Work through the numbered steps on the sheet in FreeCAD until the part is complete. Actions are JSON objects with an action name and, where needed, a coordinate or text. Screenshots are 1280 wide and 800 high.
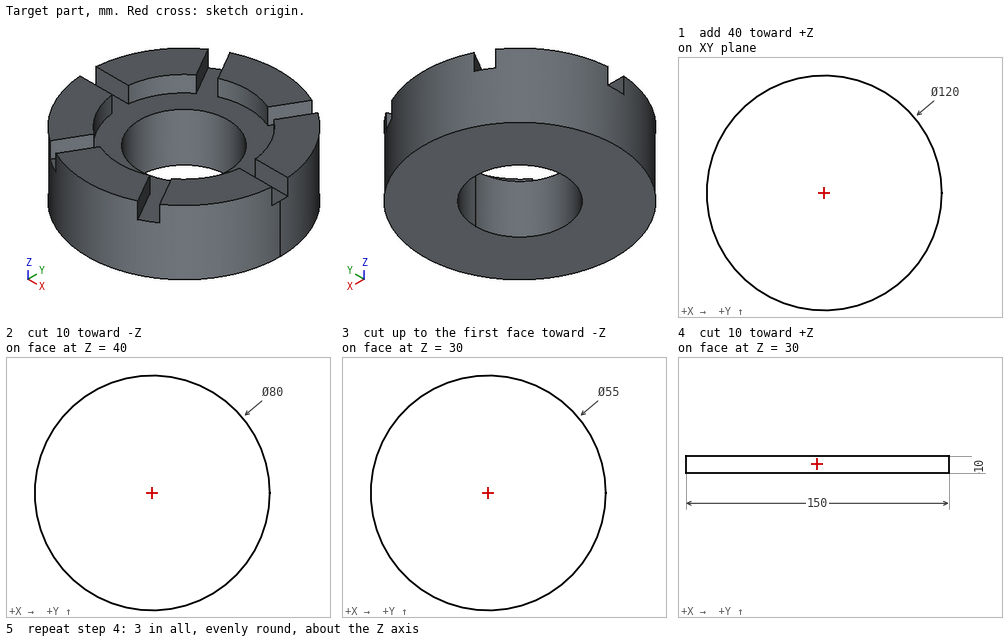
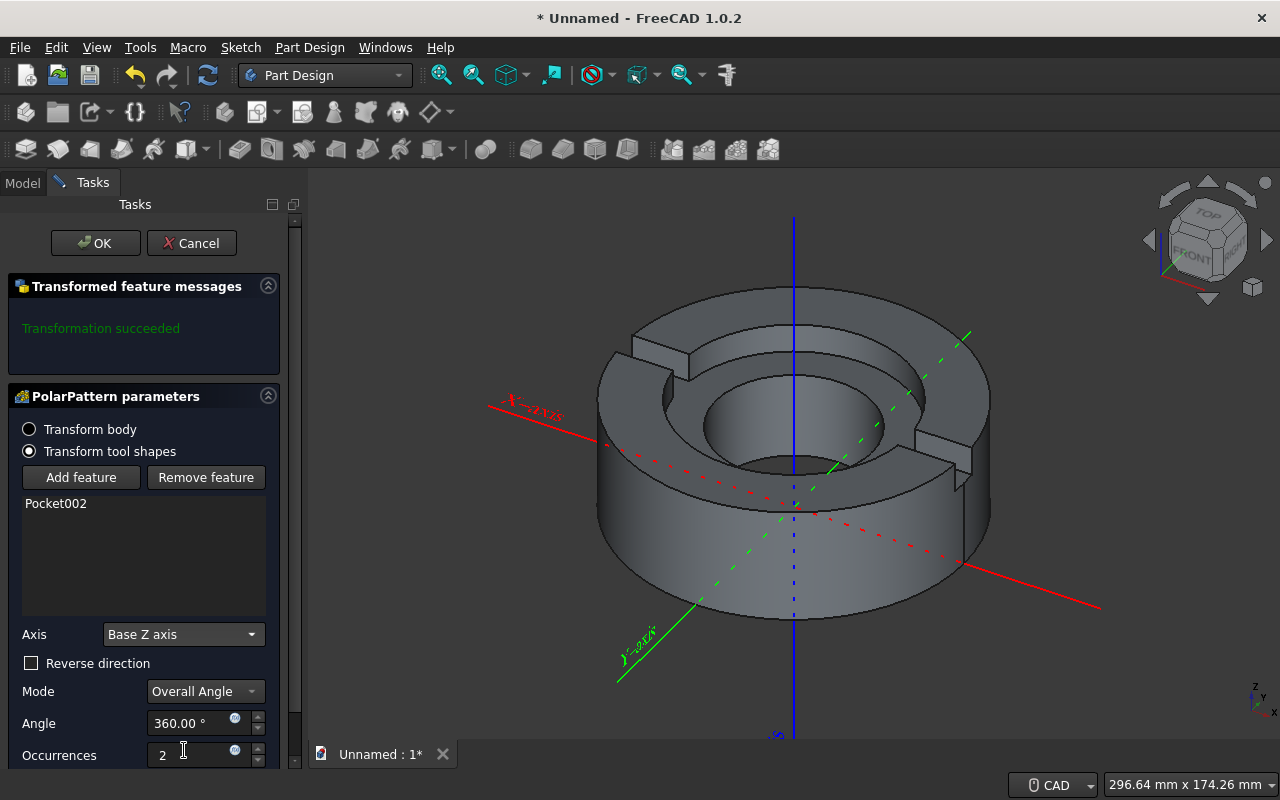
{"action": "triple_click", "coordinate": [198, 755]}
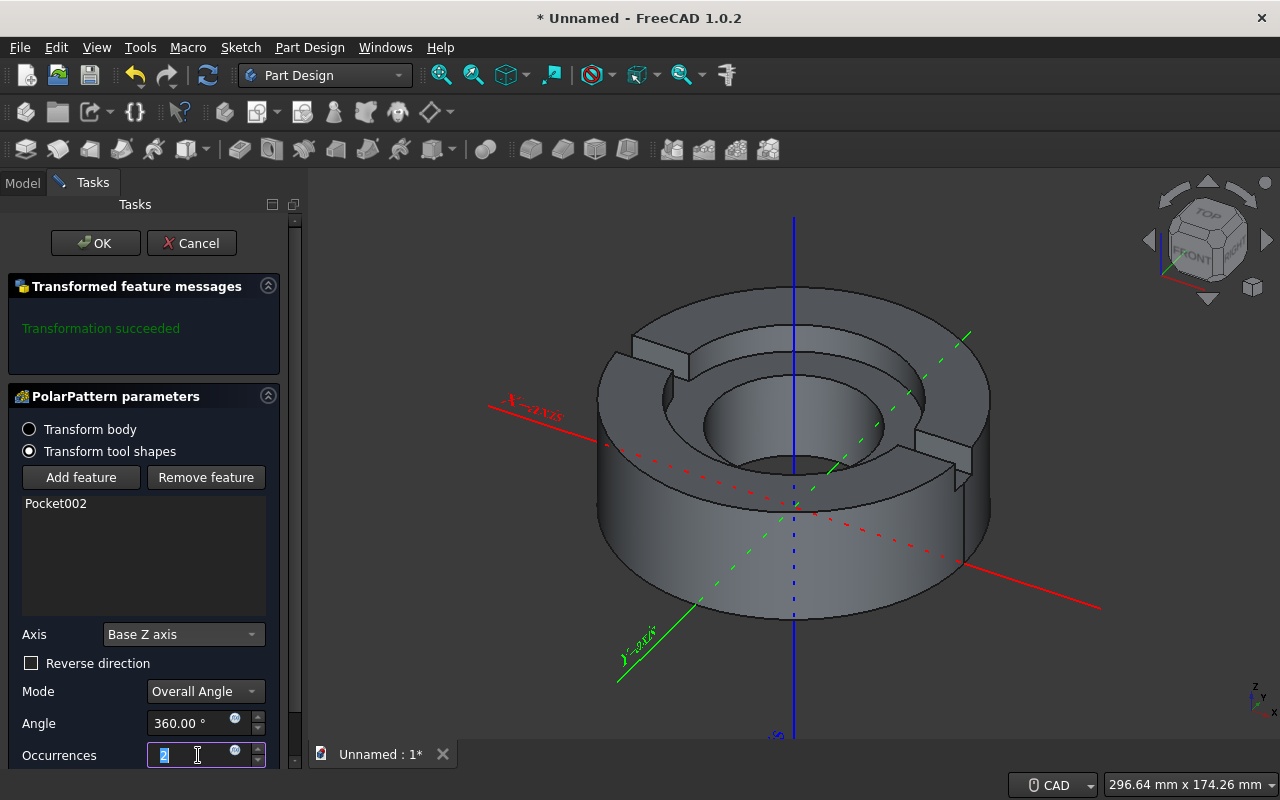
{"action": "type", "text": "3"}
{"action": "key", "text": "Tab"}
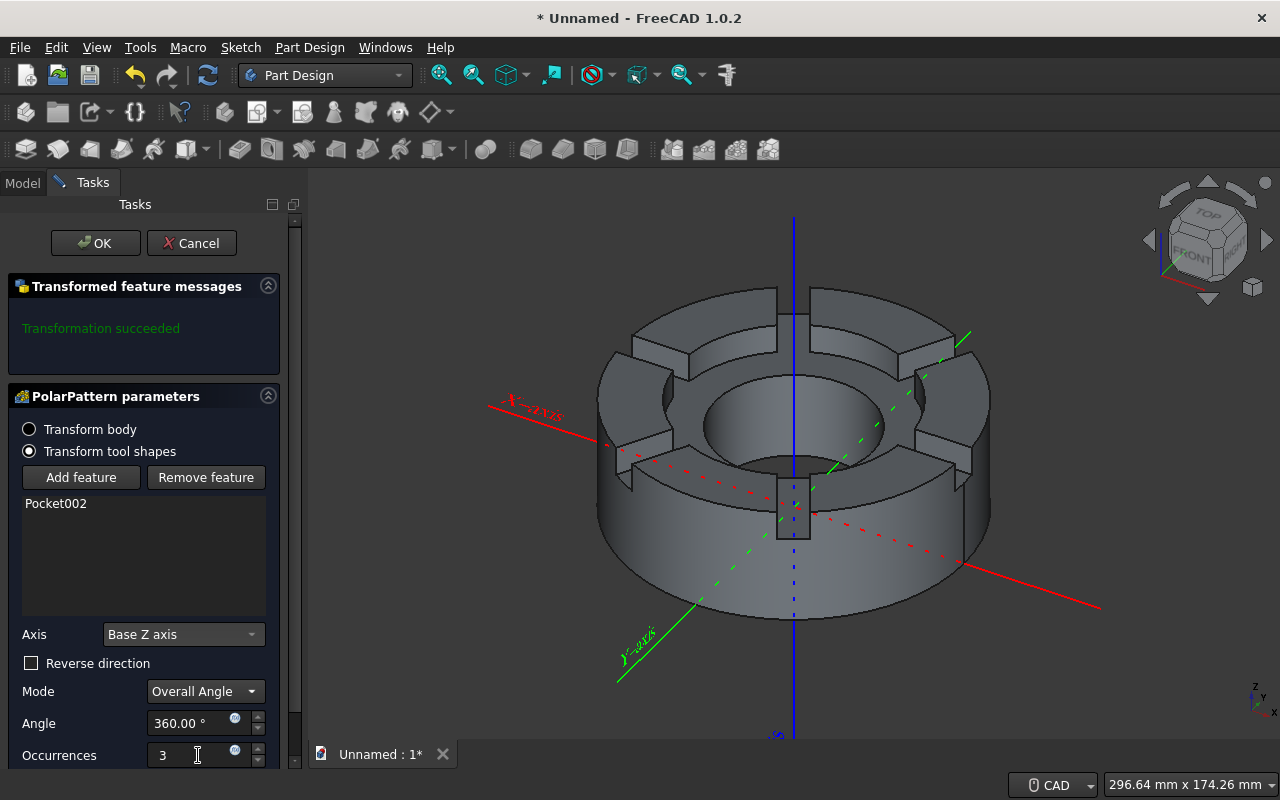
{"action": "left_click", "coordinate": [96, 243]}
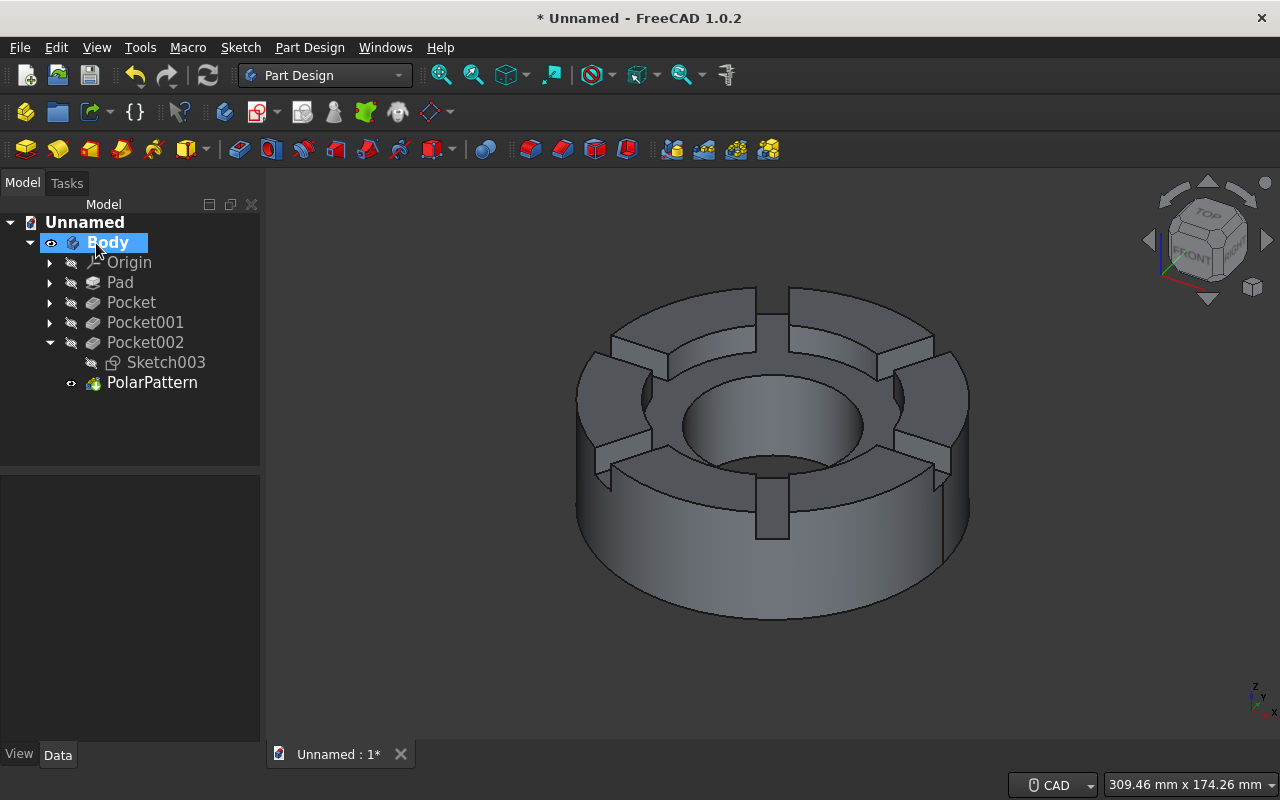
{"action": "key", "text": "0"}